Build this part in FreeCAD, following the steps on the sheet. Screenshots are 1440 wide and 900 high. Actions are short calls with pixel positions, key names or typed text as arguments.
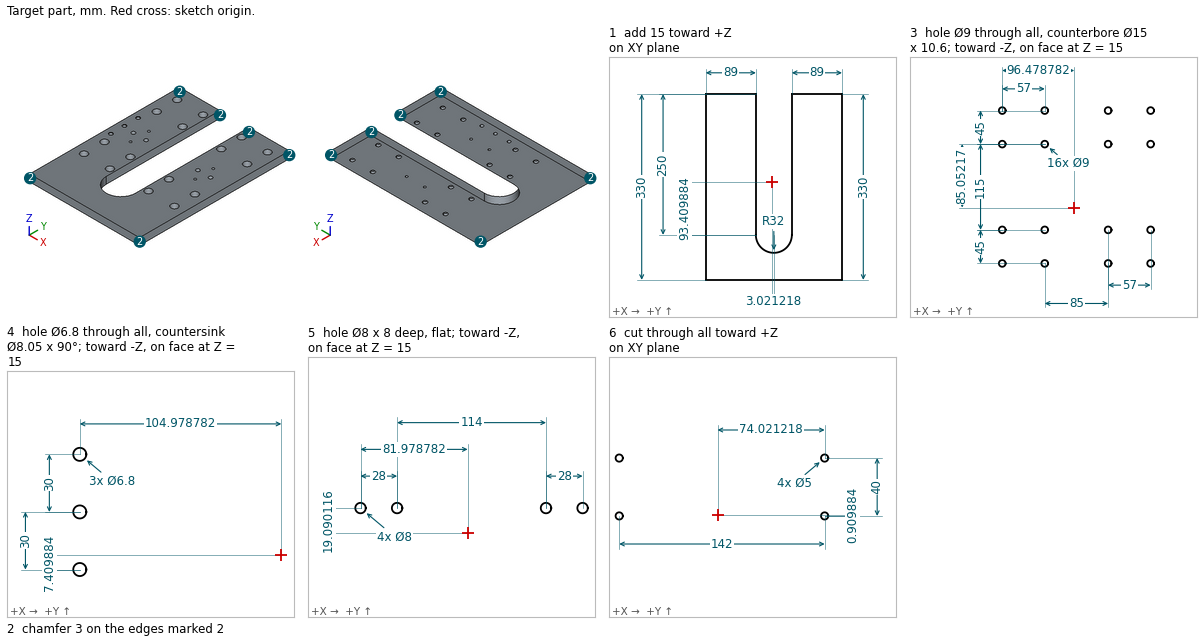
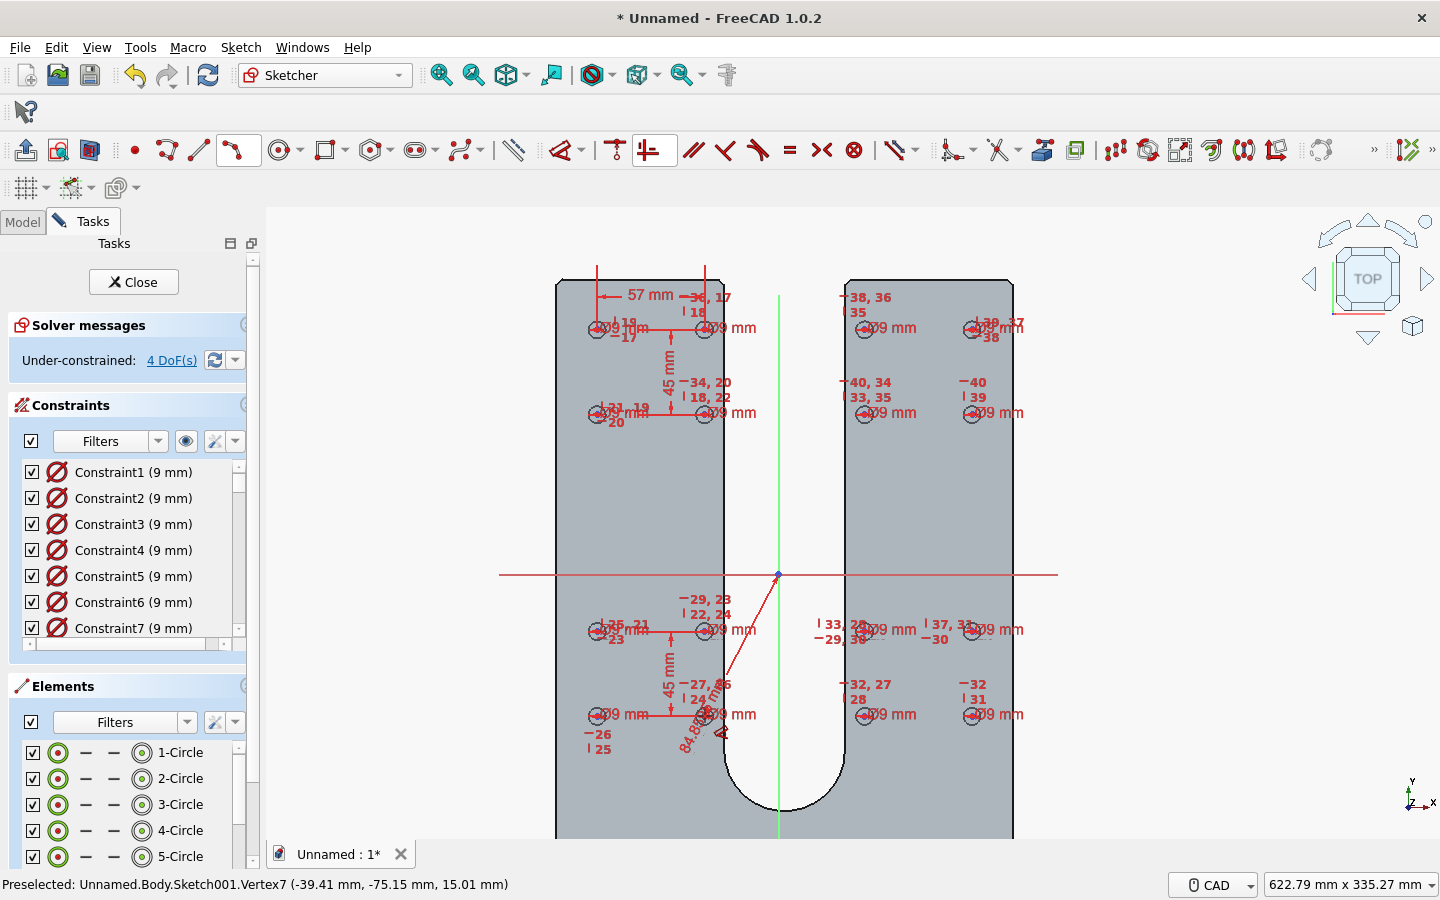
click(865, 716)
click(748, 750)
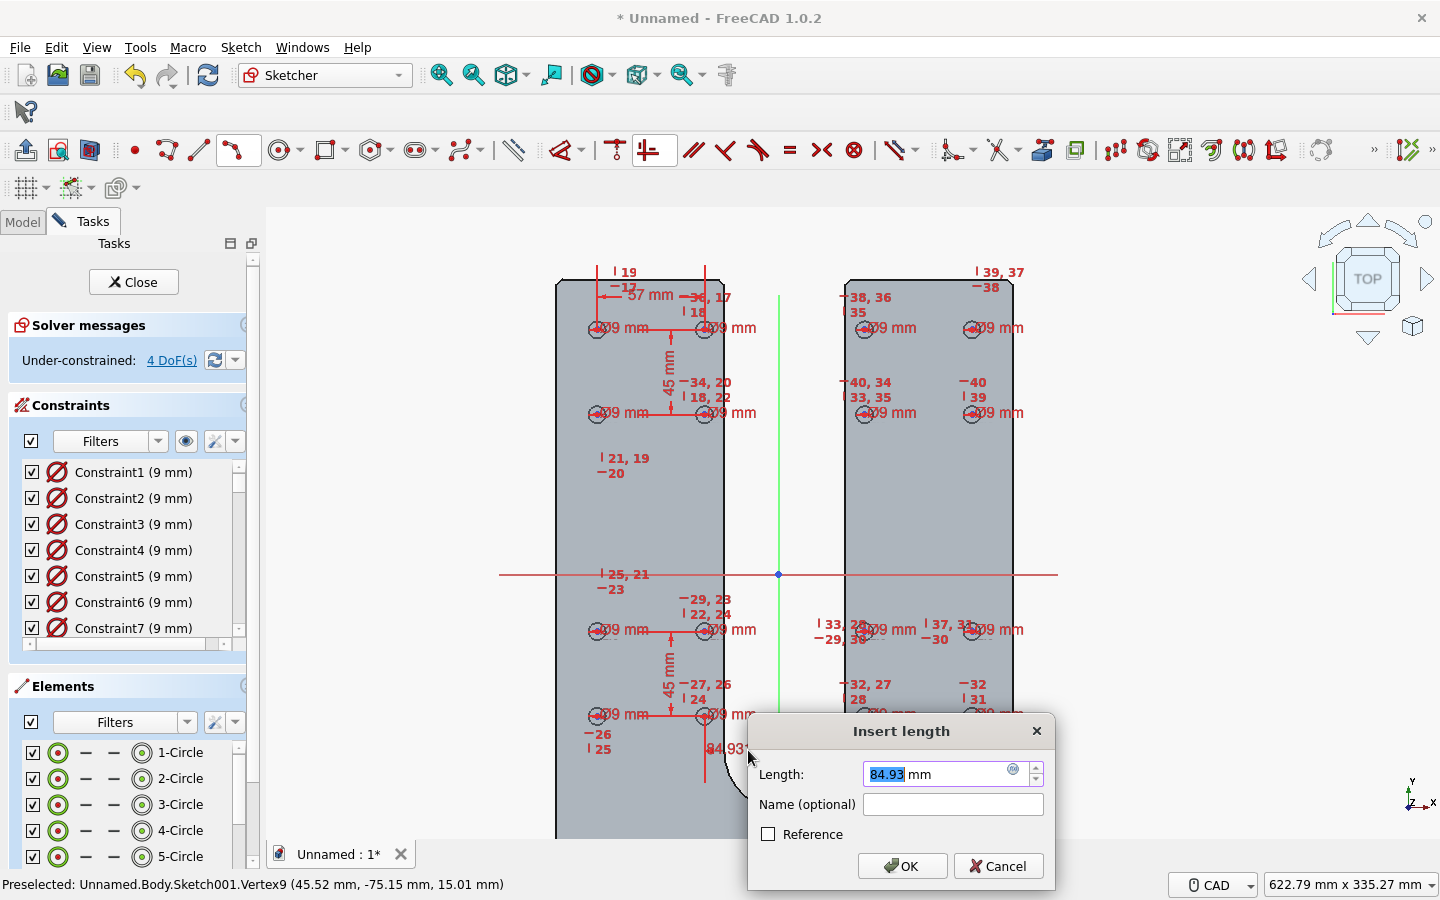
text(85)
key(Return)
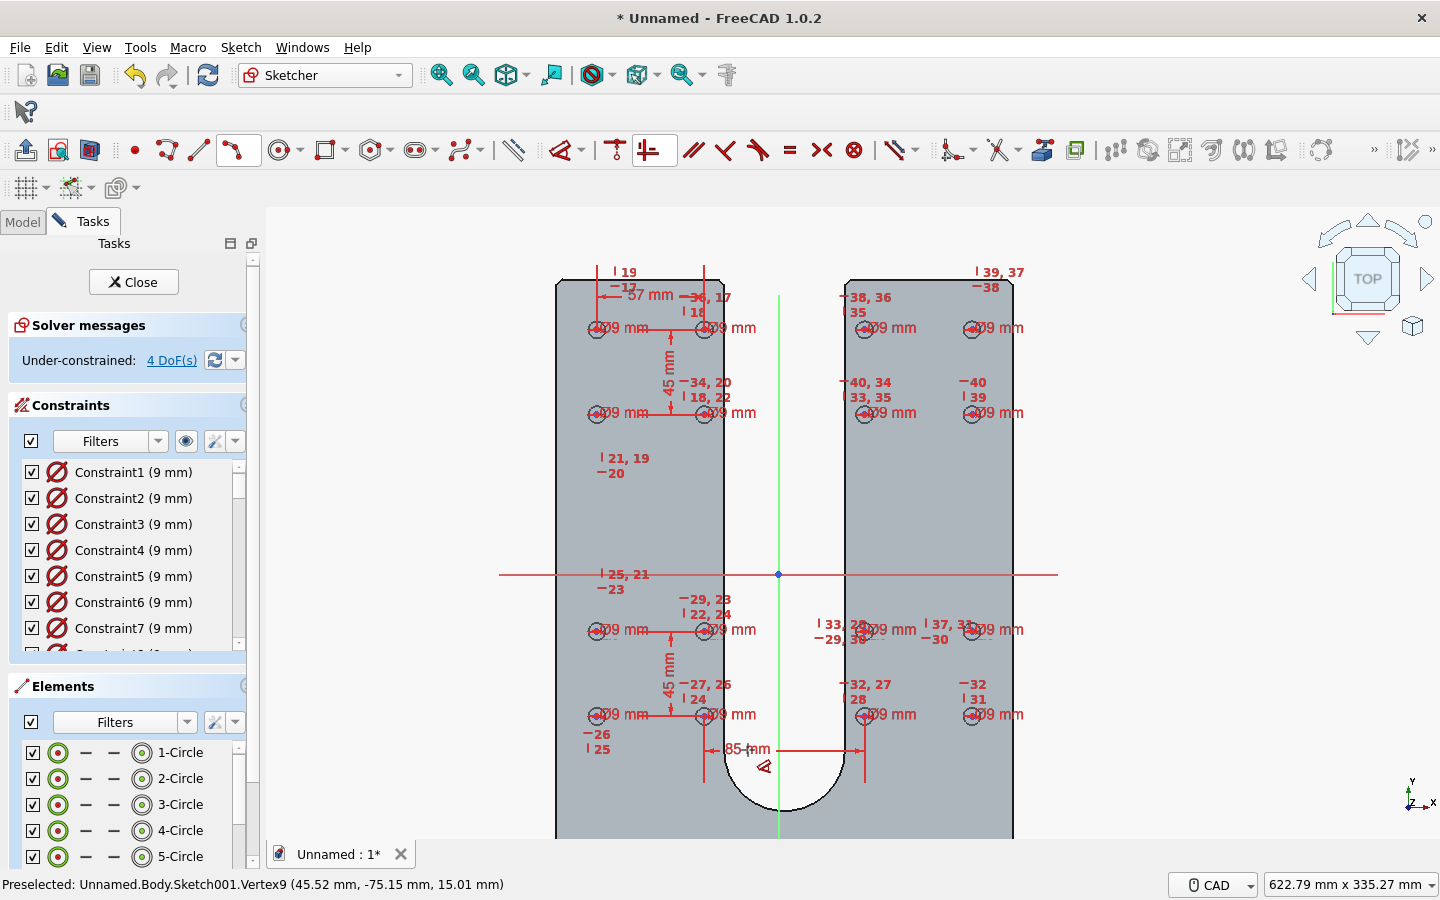
click(865, 632)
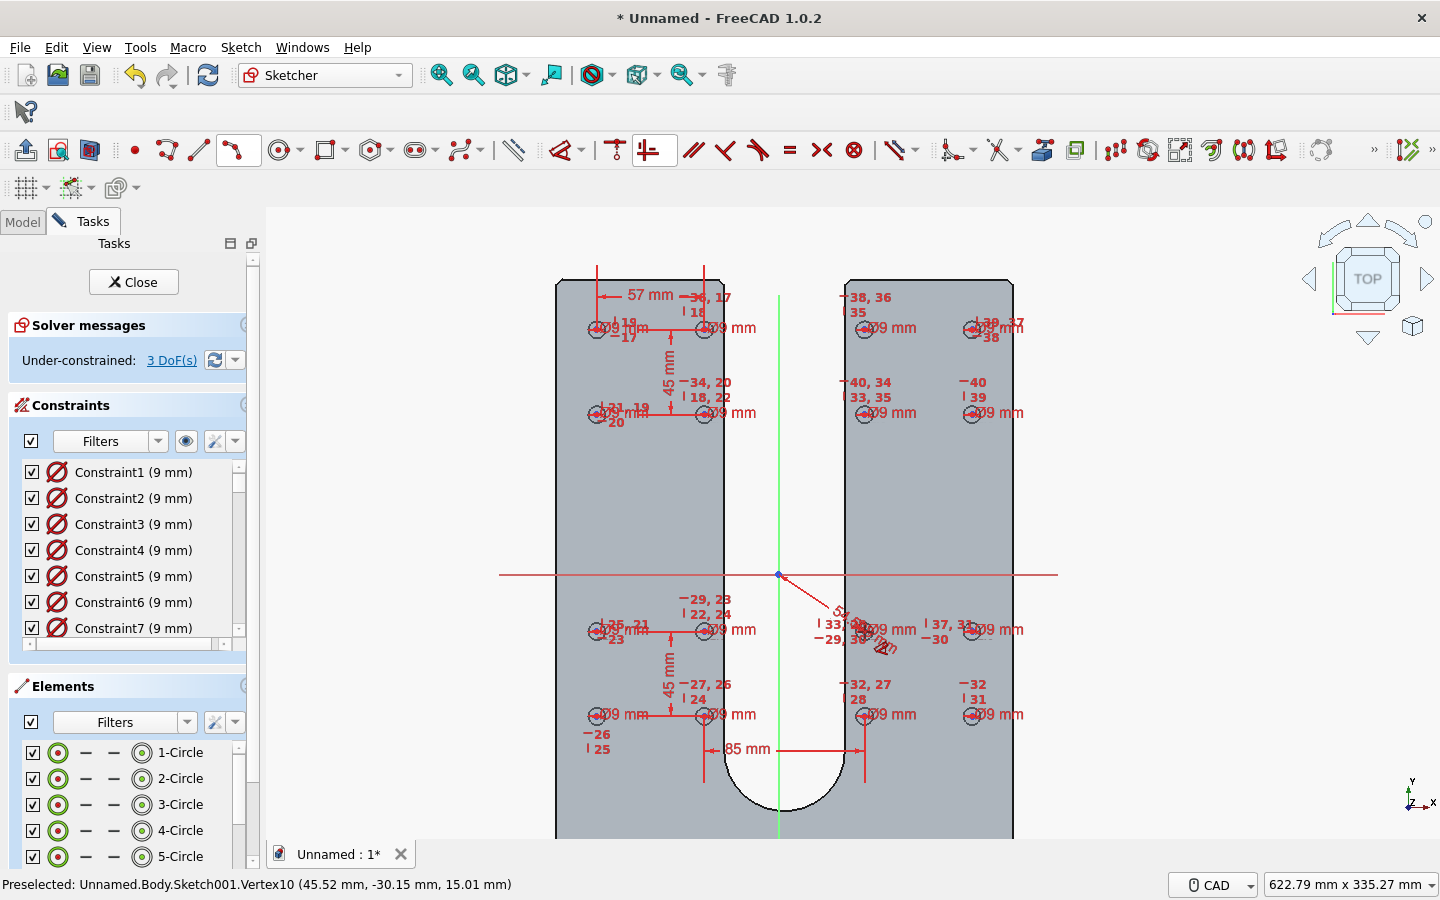
click(972, 632)
click(918, 666)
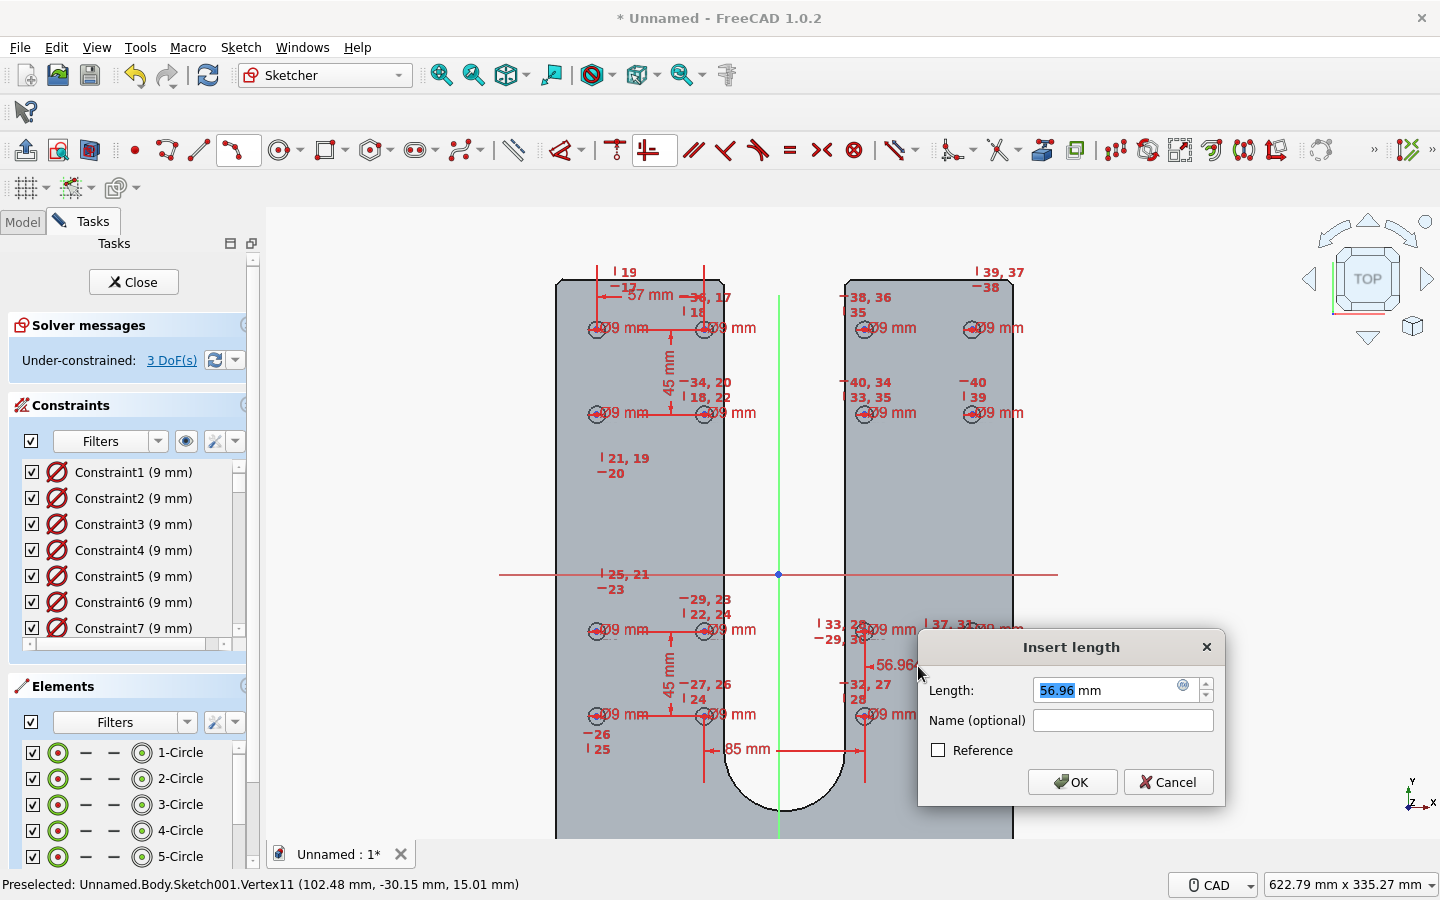
text(57)
key(Return)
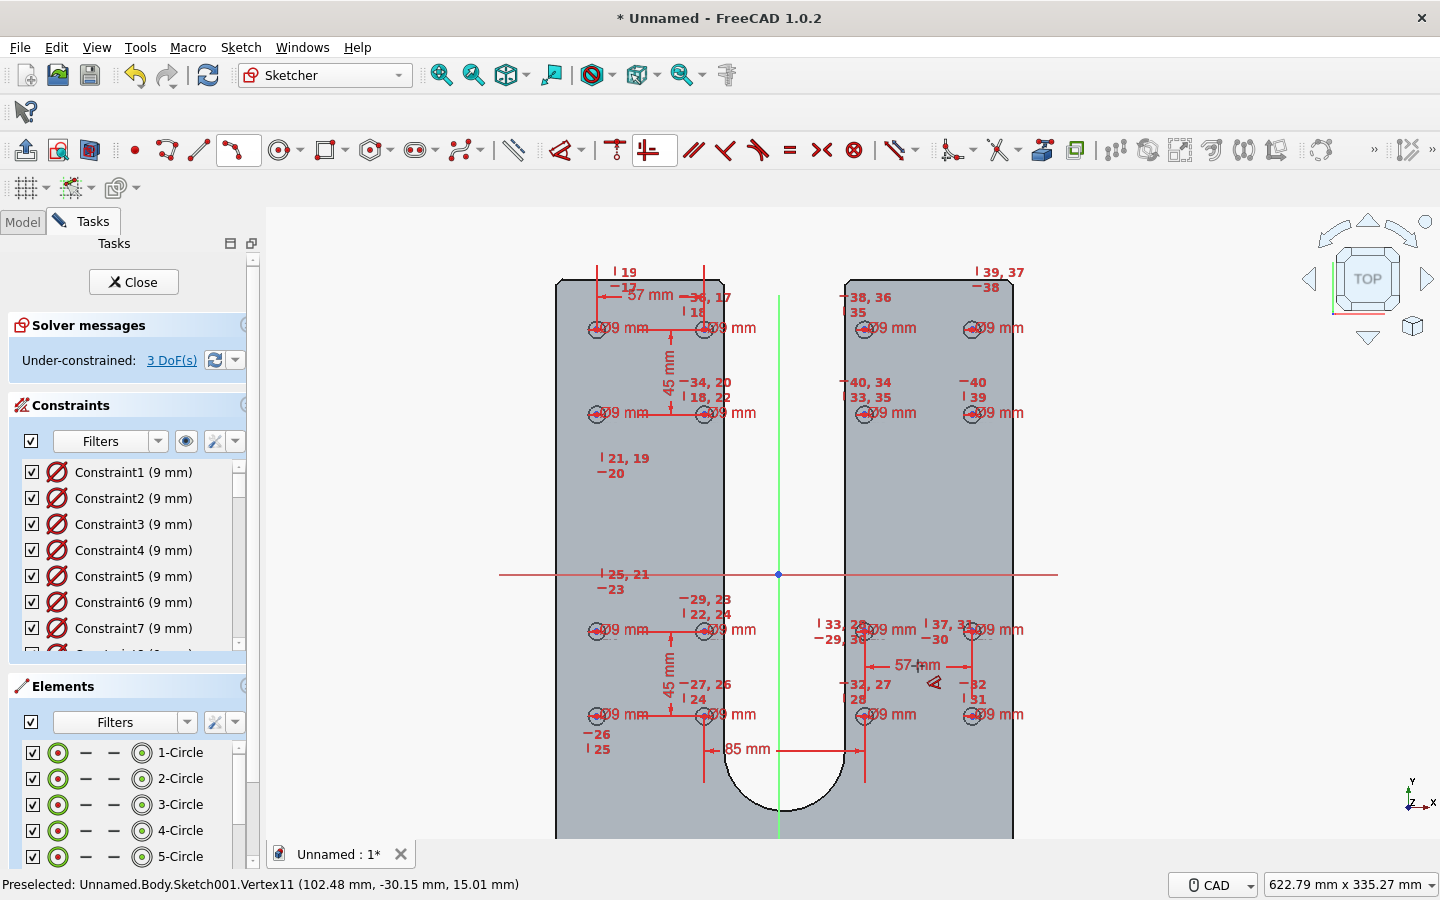
click(597, 415)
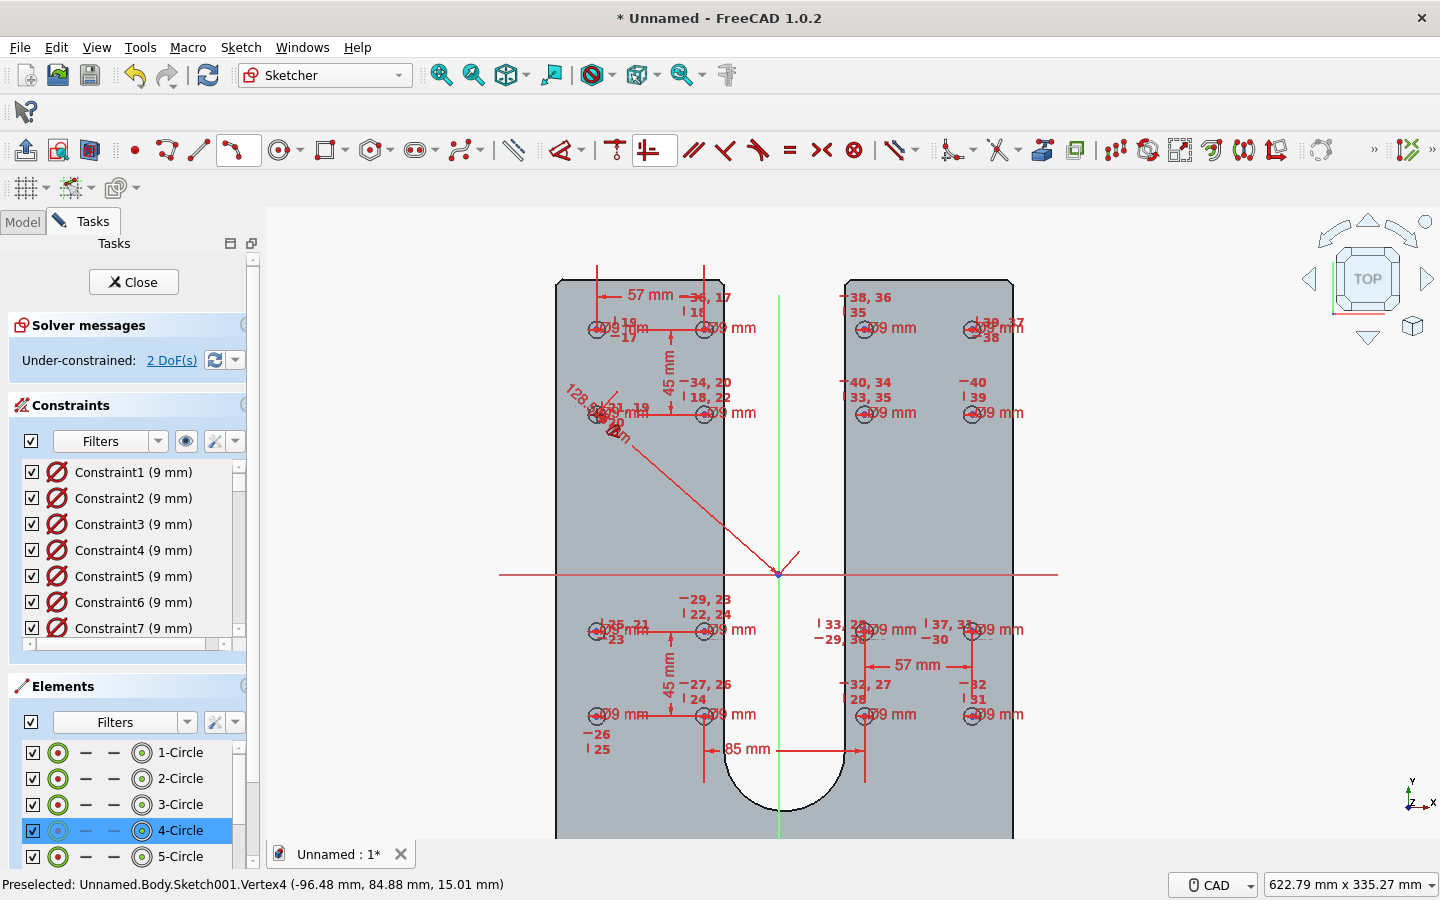
click(597, 632)
click(563, 523)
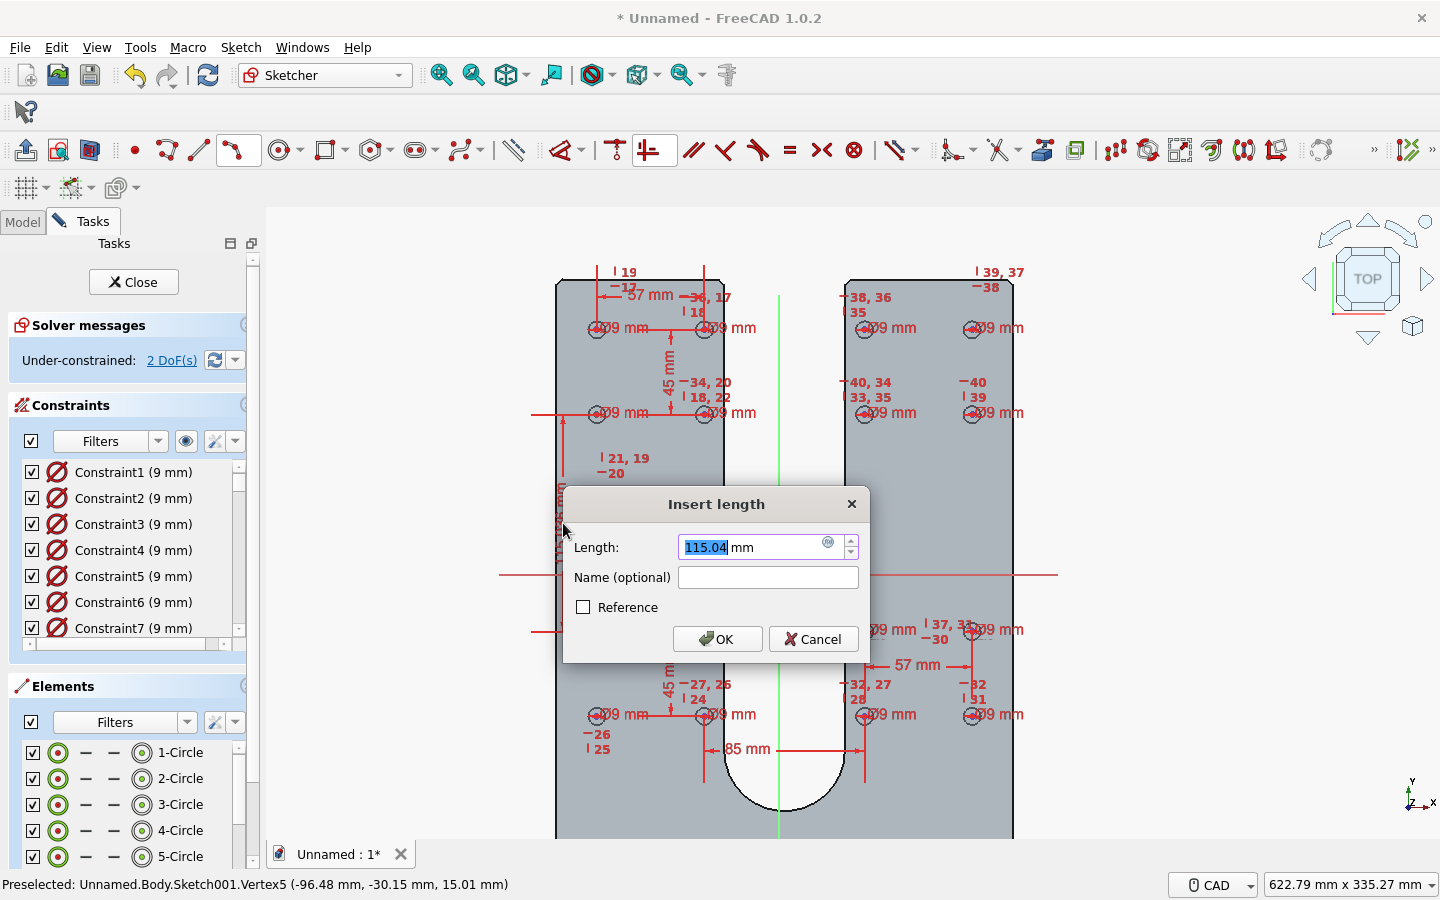
text(115)
key(Return)